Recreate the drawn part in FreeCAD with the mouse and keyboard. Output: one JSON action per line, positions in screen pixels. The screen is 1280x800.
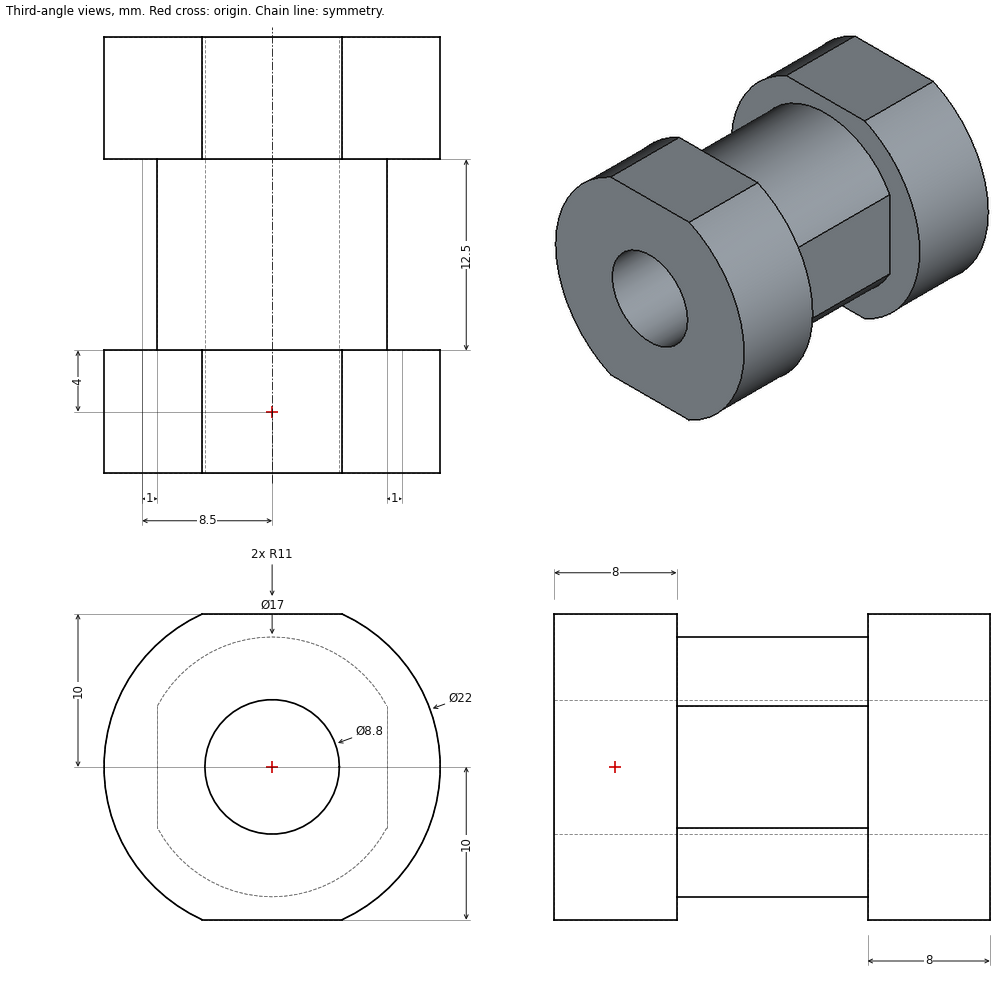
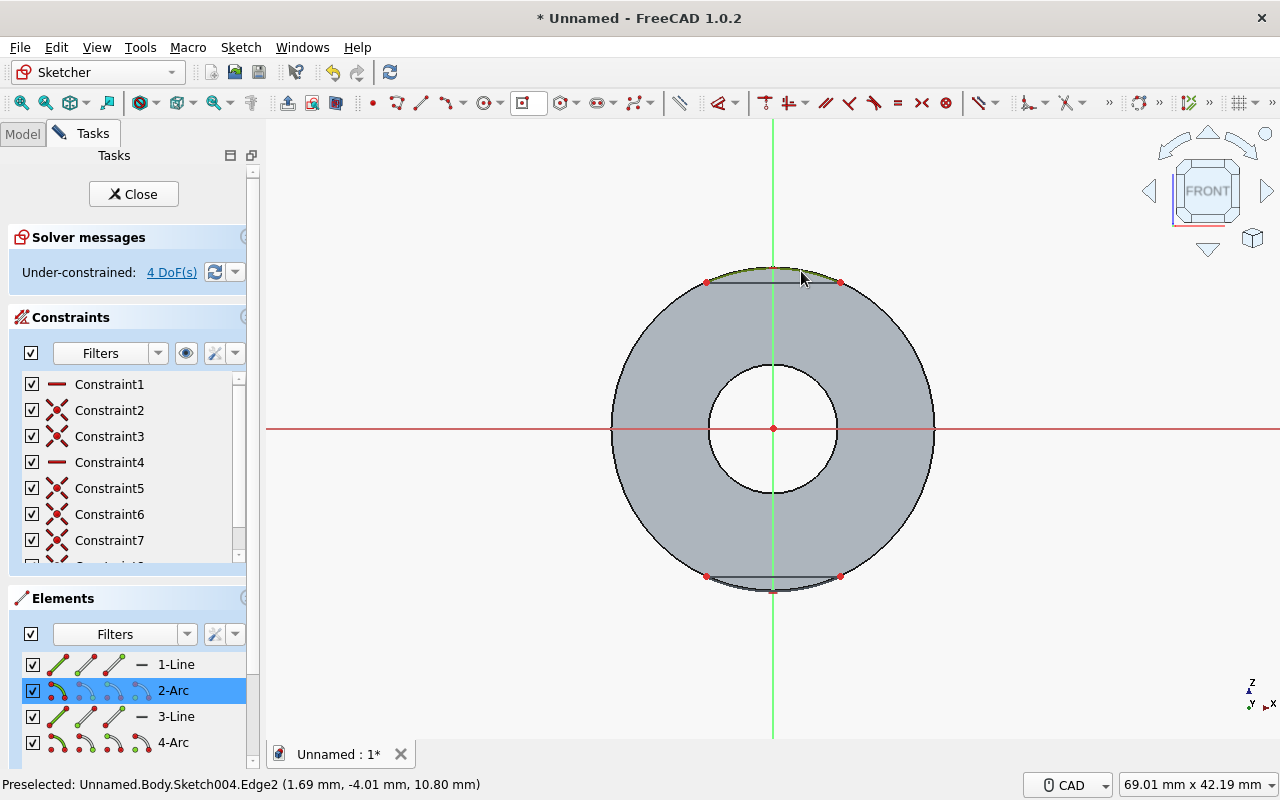
{"action": "left_click", "coordinate": [746, 589]}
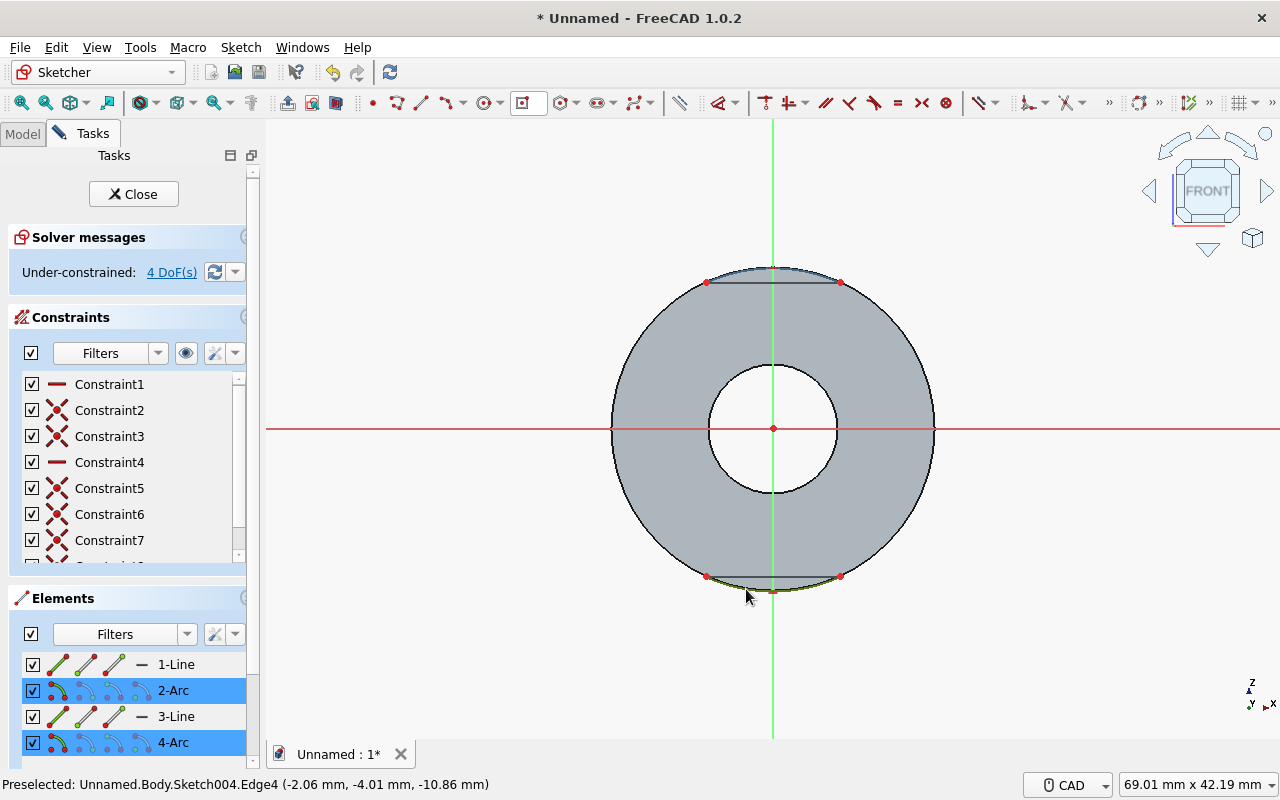
{"action": "key", "text": "e"}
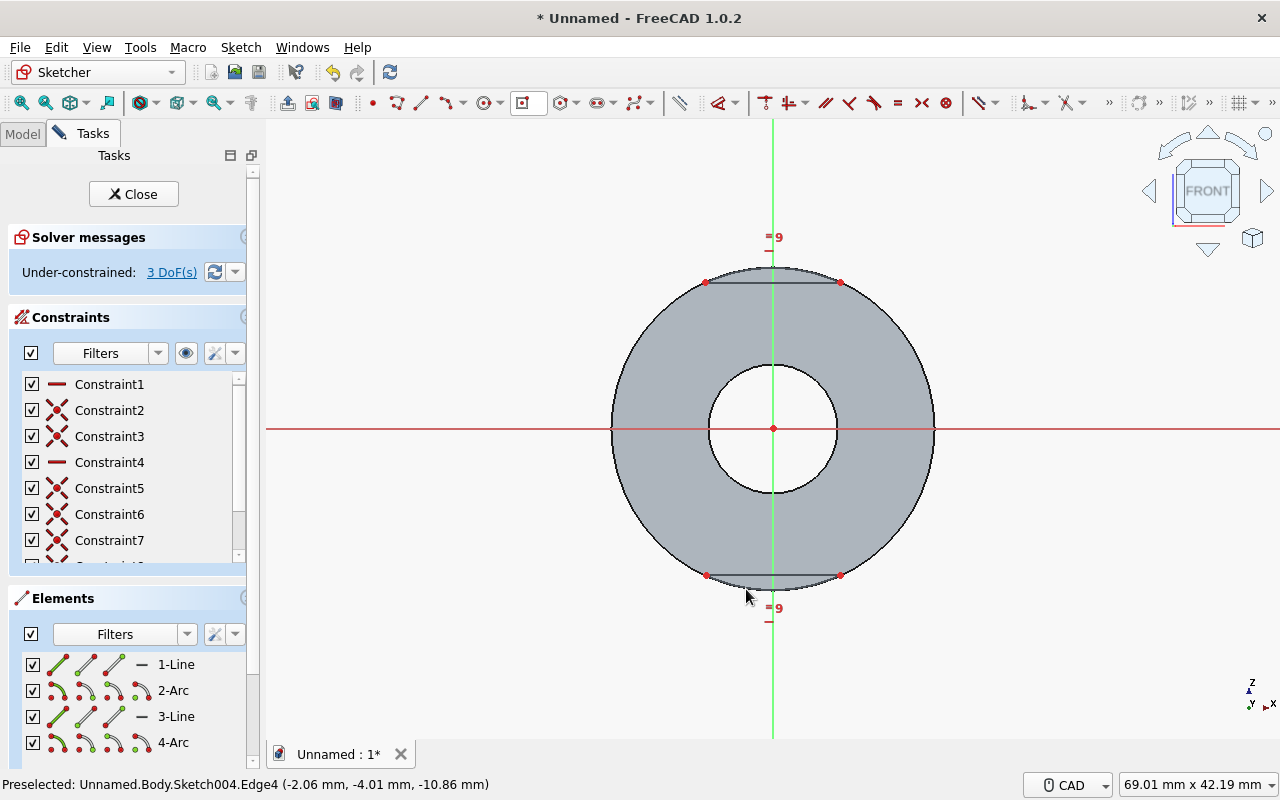
{"action": "left_click", "coordinate": [801, 270]}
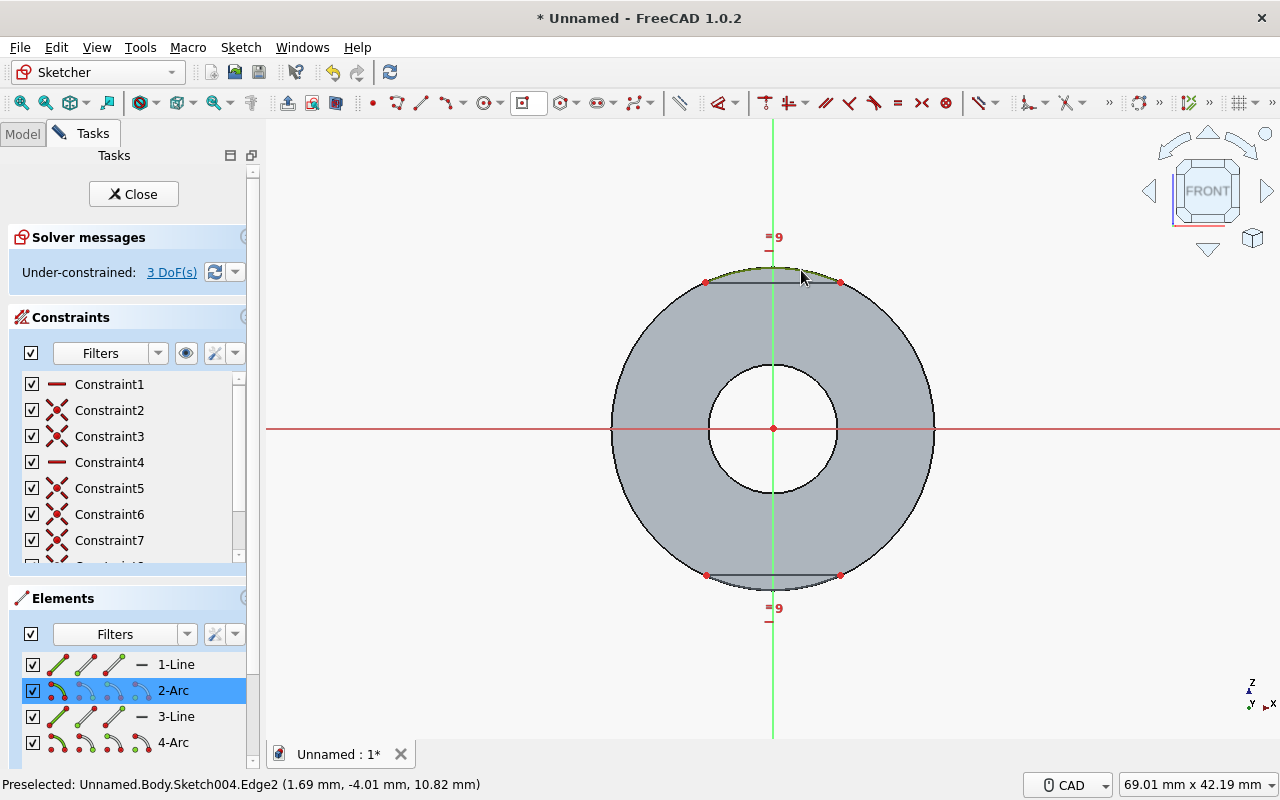
{"action": "key", "text": "k r"}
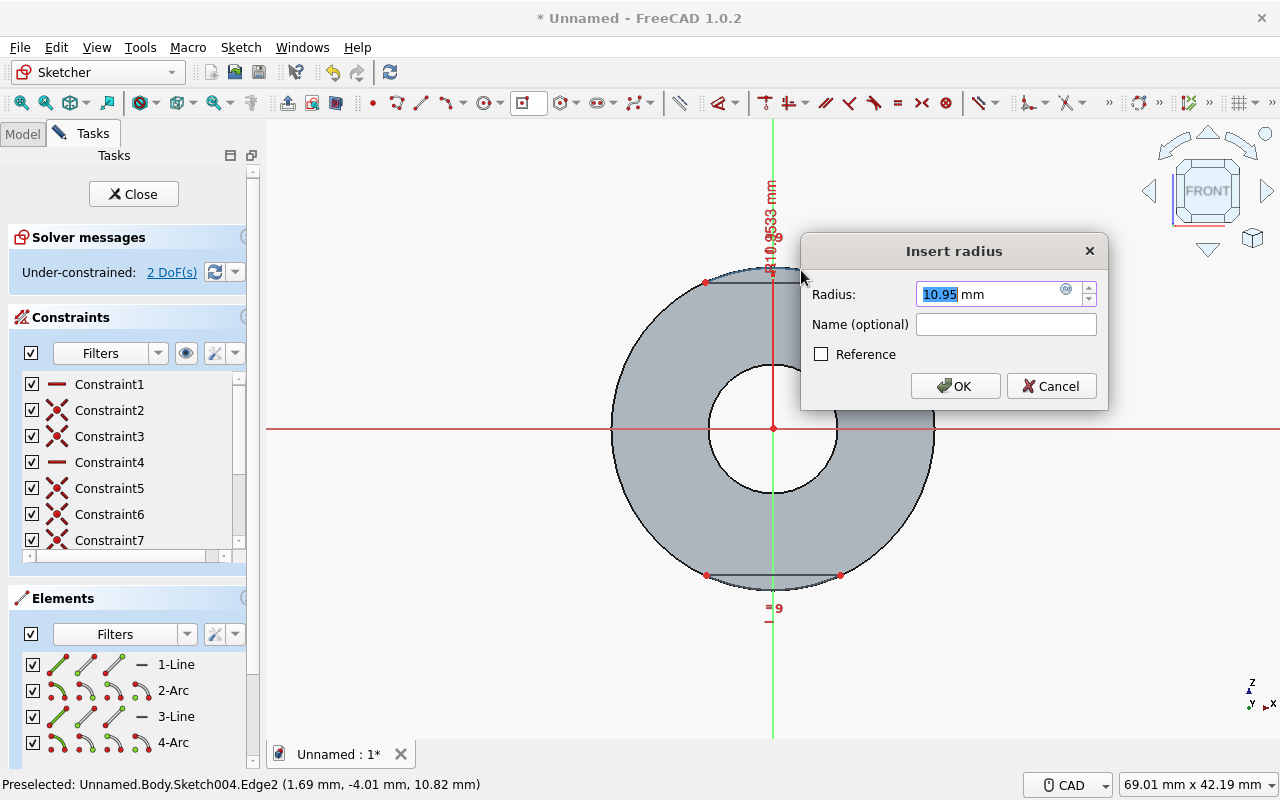
{"action": "type", "text": "11"}
{"action": "key", "text": "Return"}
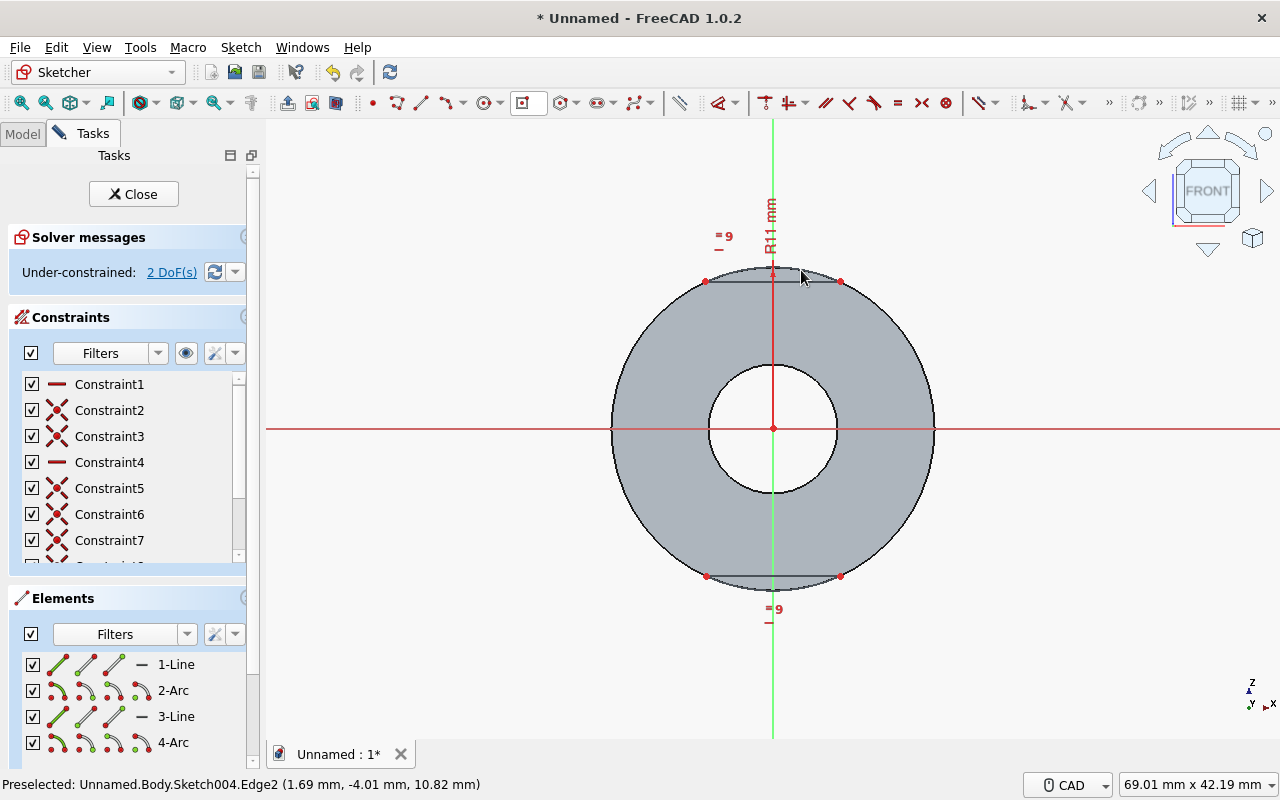
{"action": "left_click", "coordinate": [706, 282]}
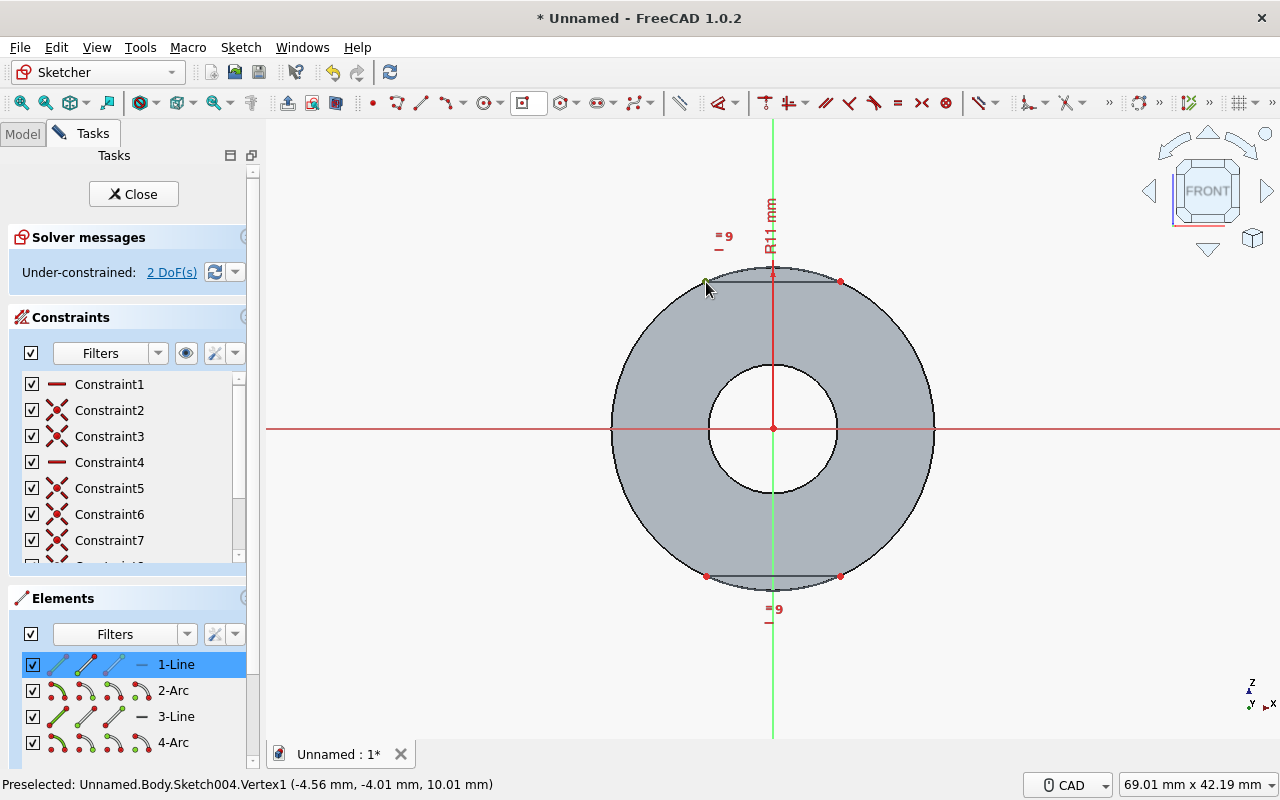
{"action": "key", "text": "i"}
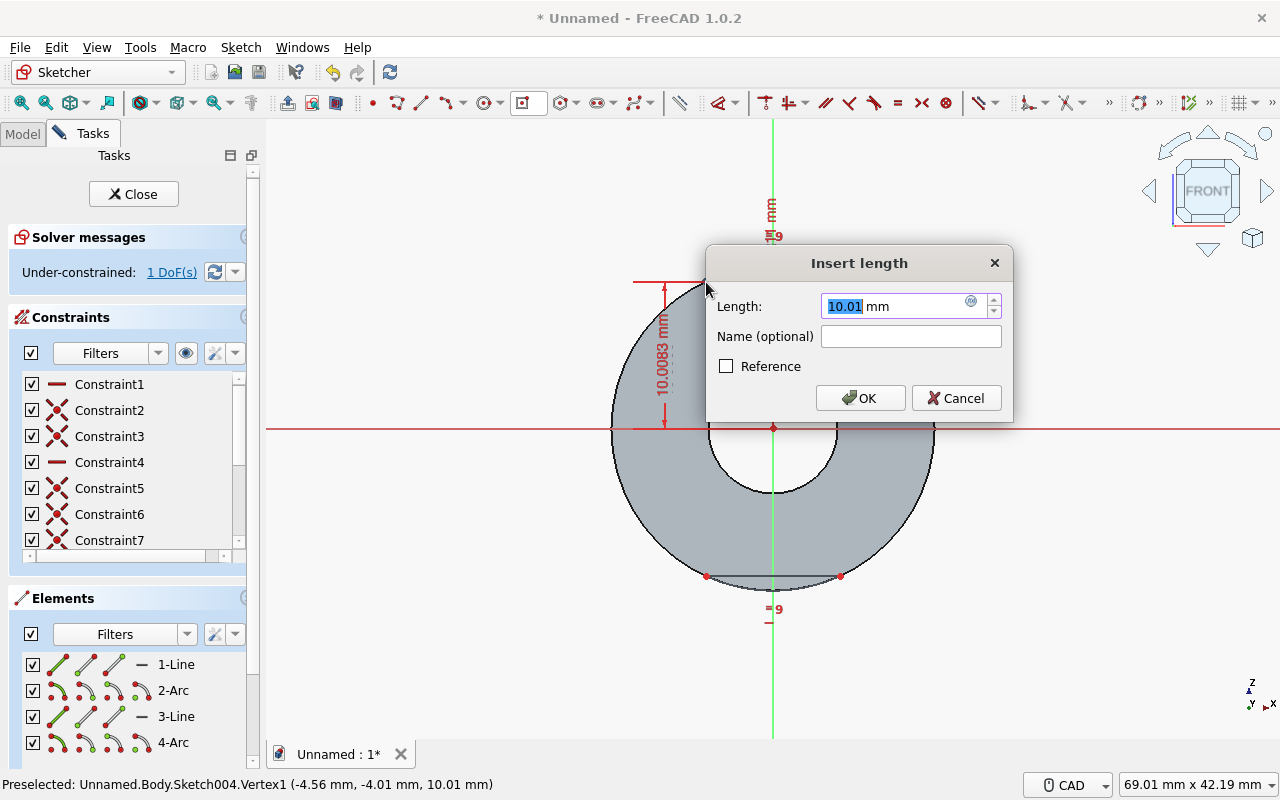
{"action": "type", "text": "10"}
{"action": "key", "text": "Return"}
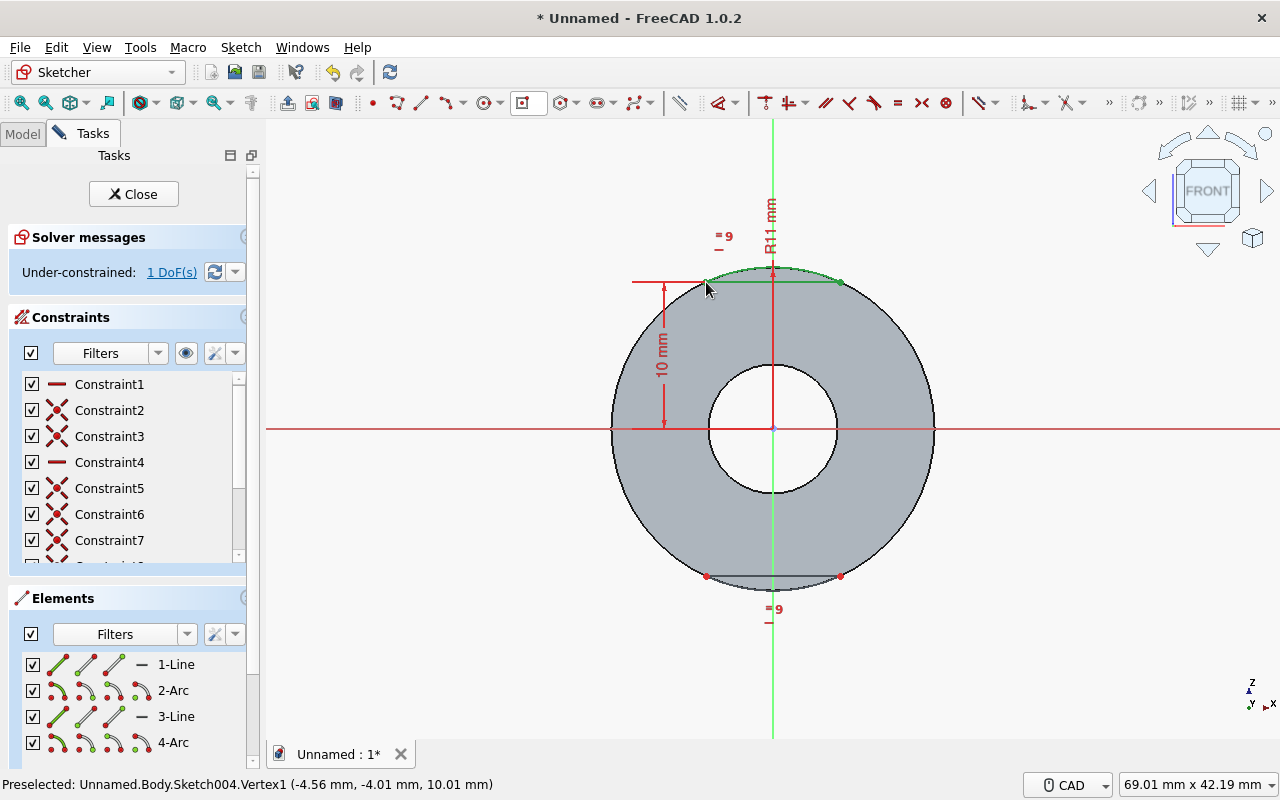
{"action": "left_click", "coordinate": [840, 576]}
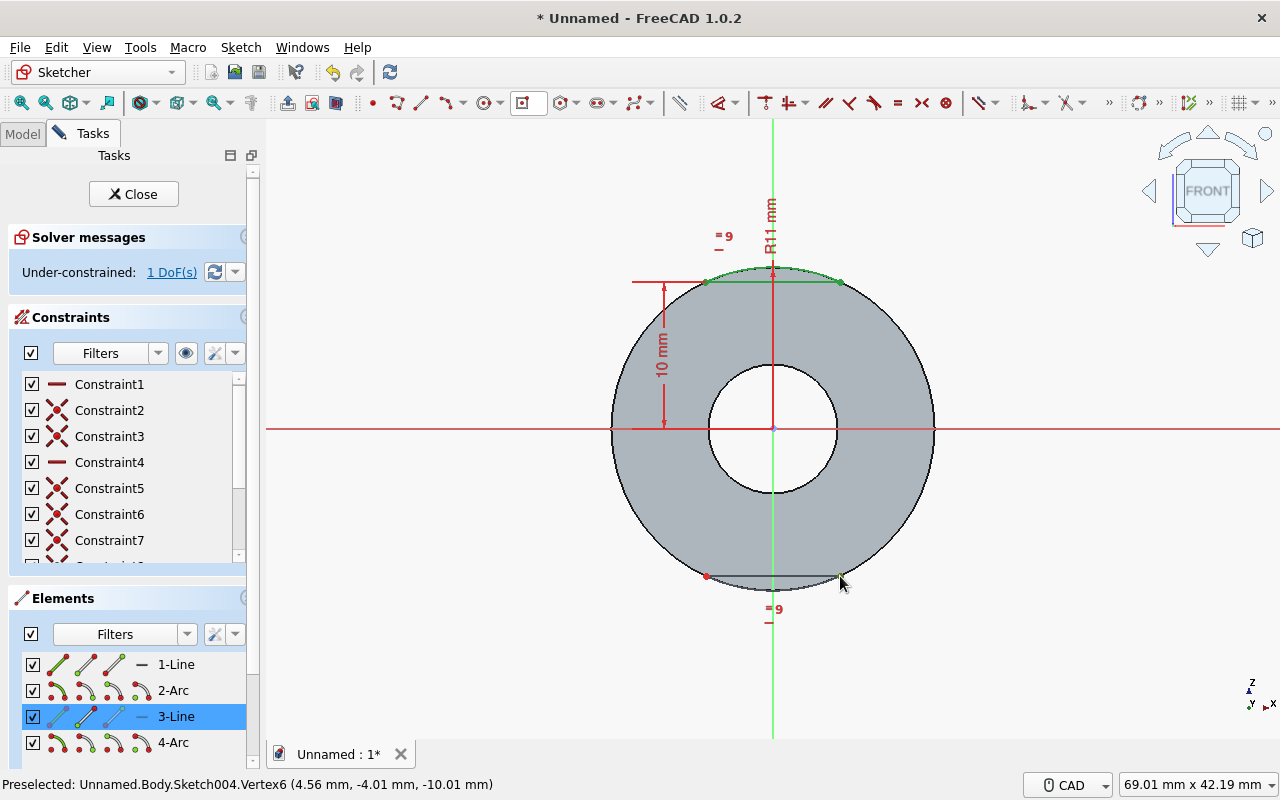
{"action": "key", "text": "i"}